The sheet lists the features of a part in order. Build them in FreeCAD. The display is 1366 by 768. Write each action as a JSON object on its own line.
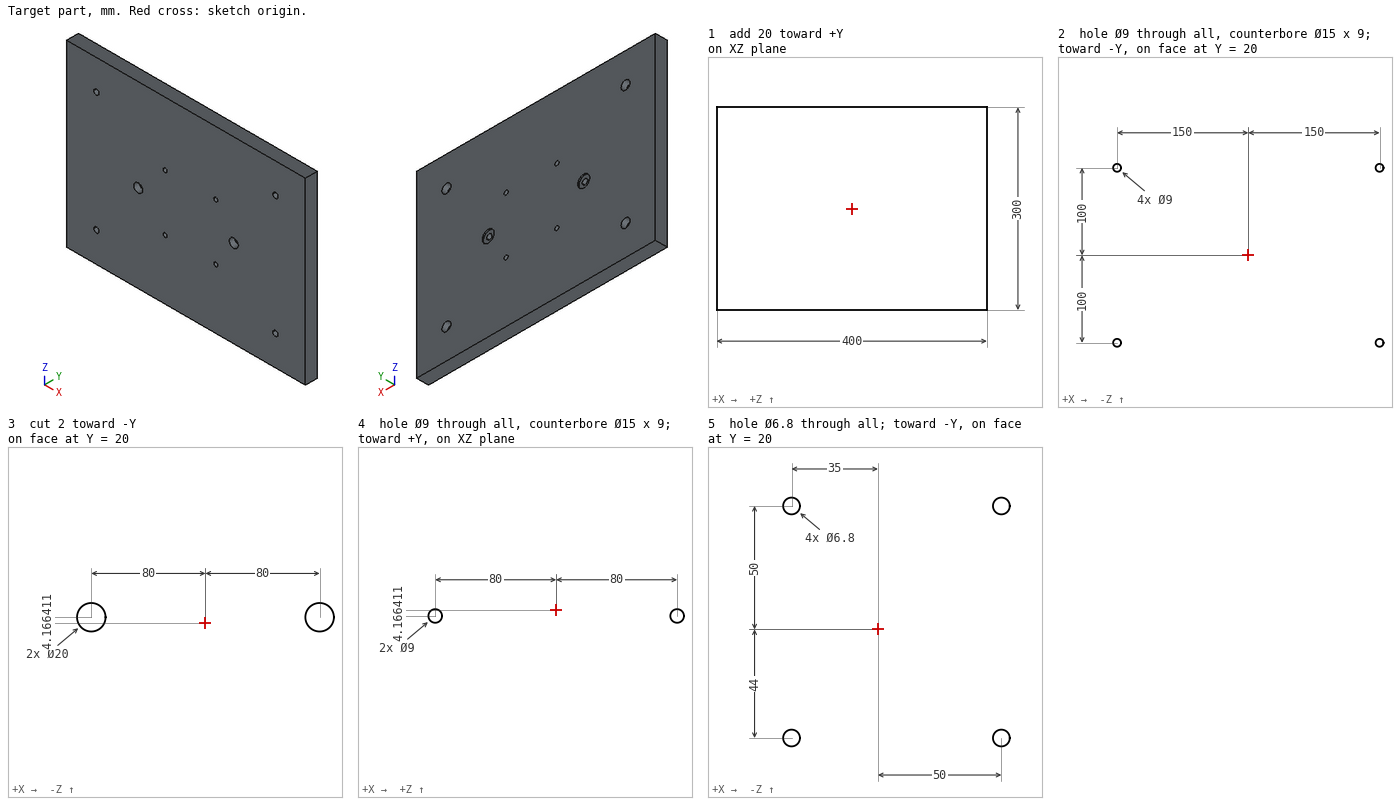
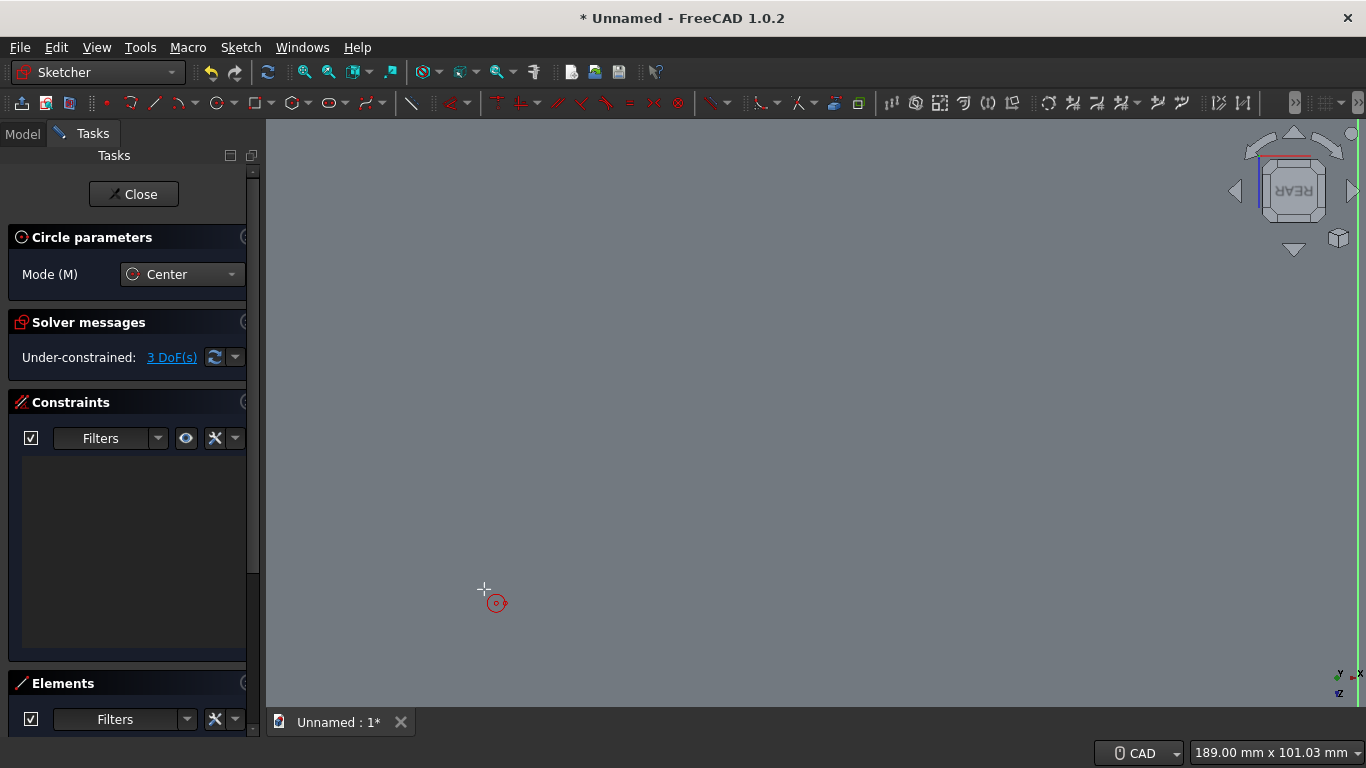
{"action": "left_click", "coordinate": [485, 586]}
{"action": "left_click", "coordinate": [503, 568]}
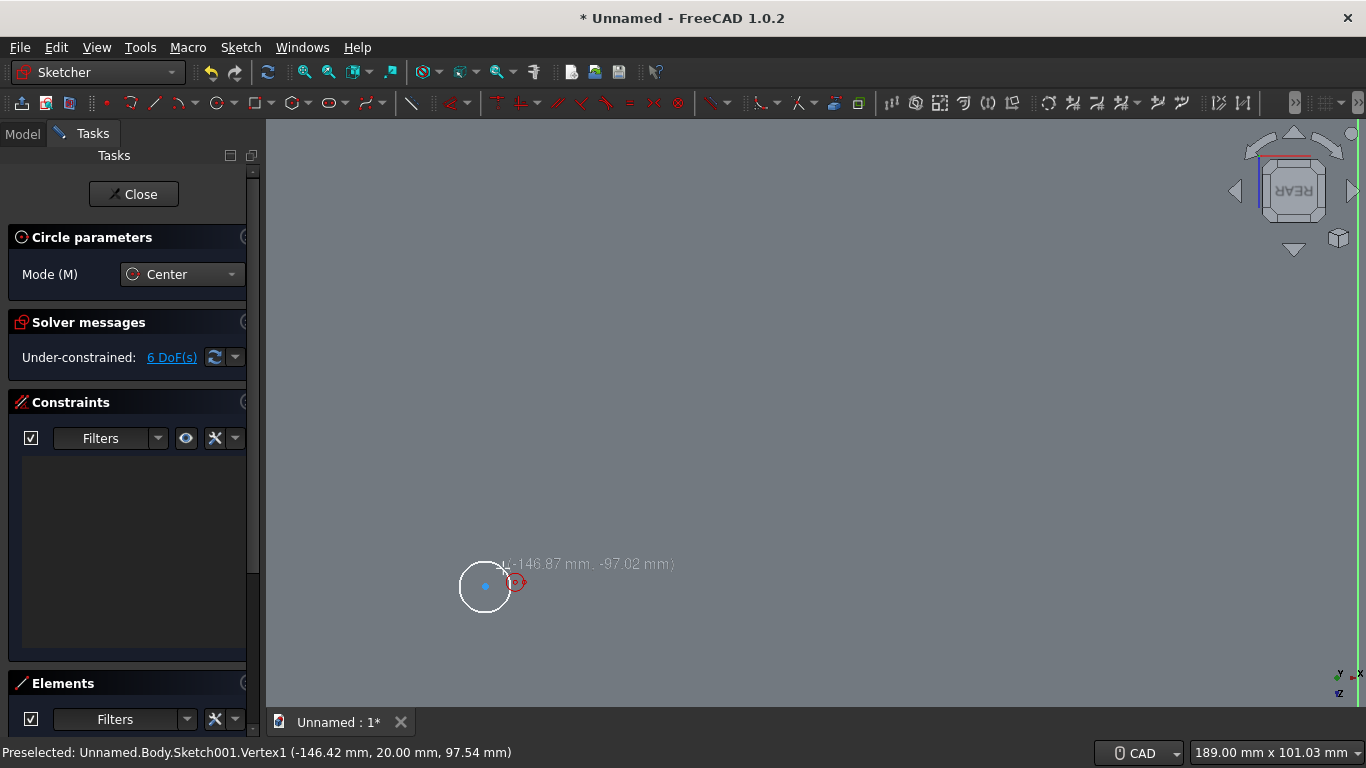
{"action": "scroll", "coordinate": [484, 589], "scroll_direction": "down", "scroll_amount": 6}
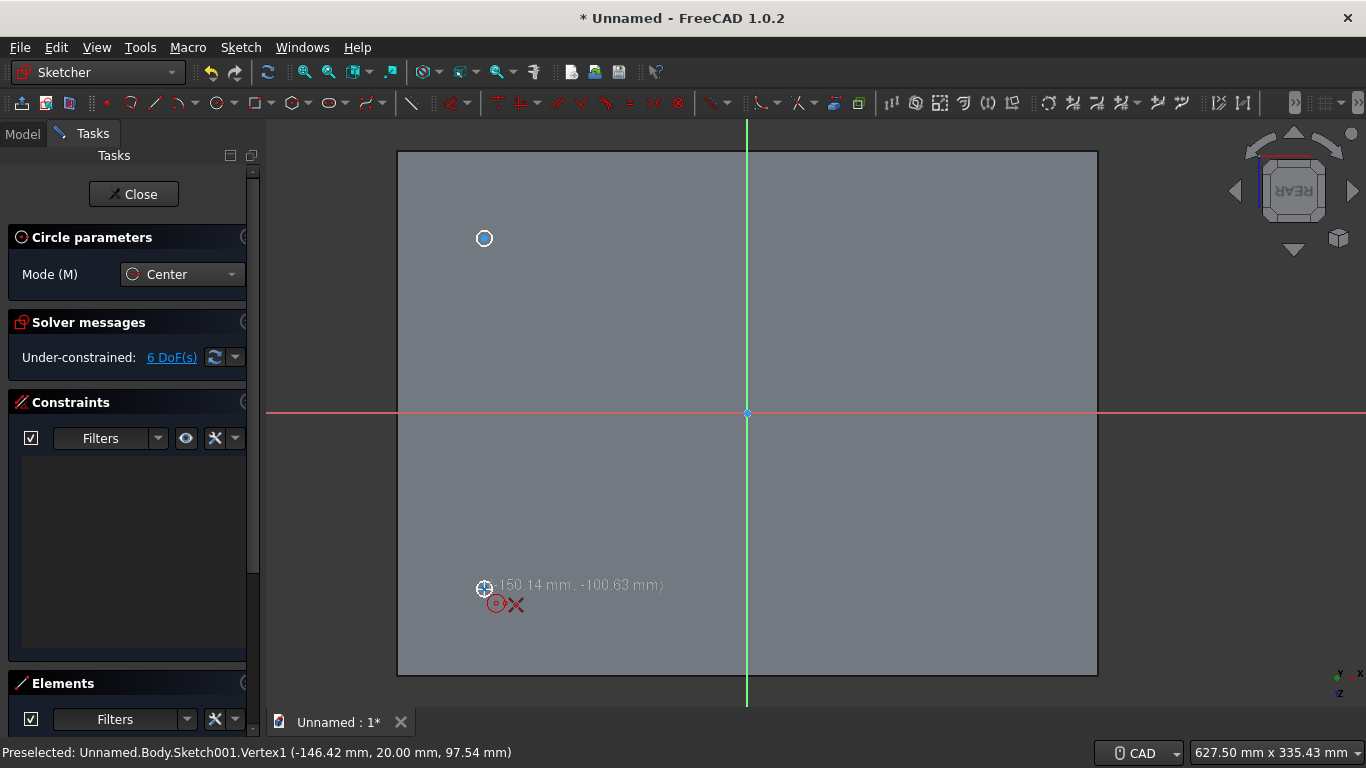
{"action": "scroll", "coordinate": [1010, 238], "scroll_direction": "up", "scroll_amount": 6}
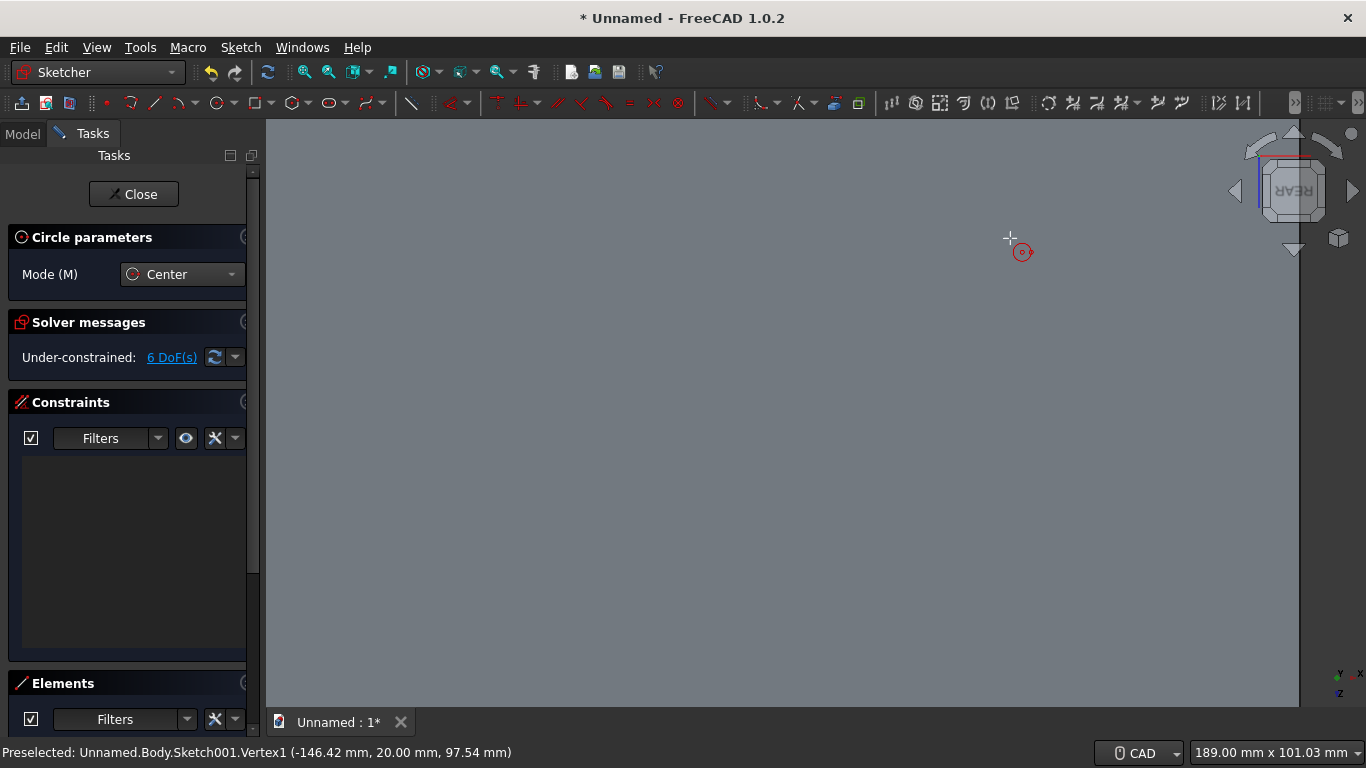
{"action": "left_click", "coordinate": [1009, 238]}
{"action": "left_click", "coordinate": [1028, 220]}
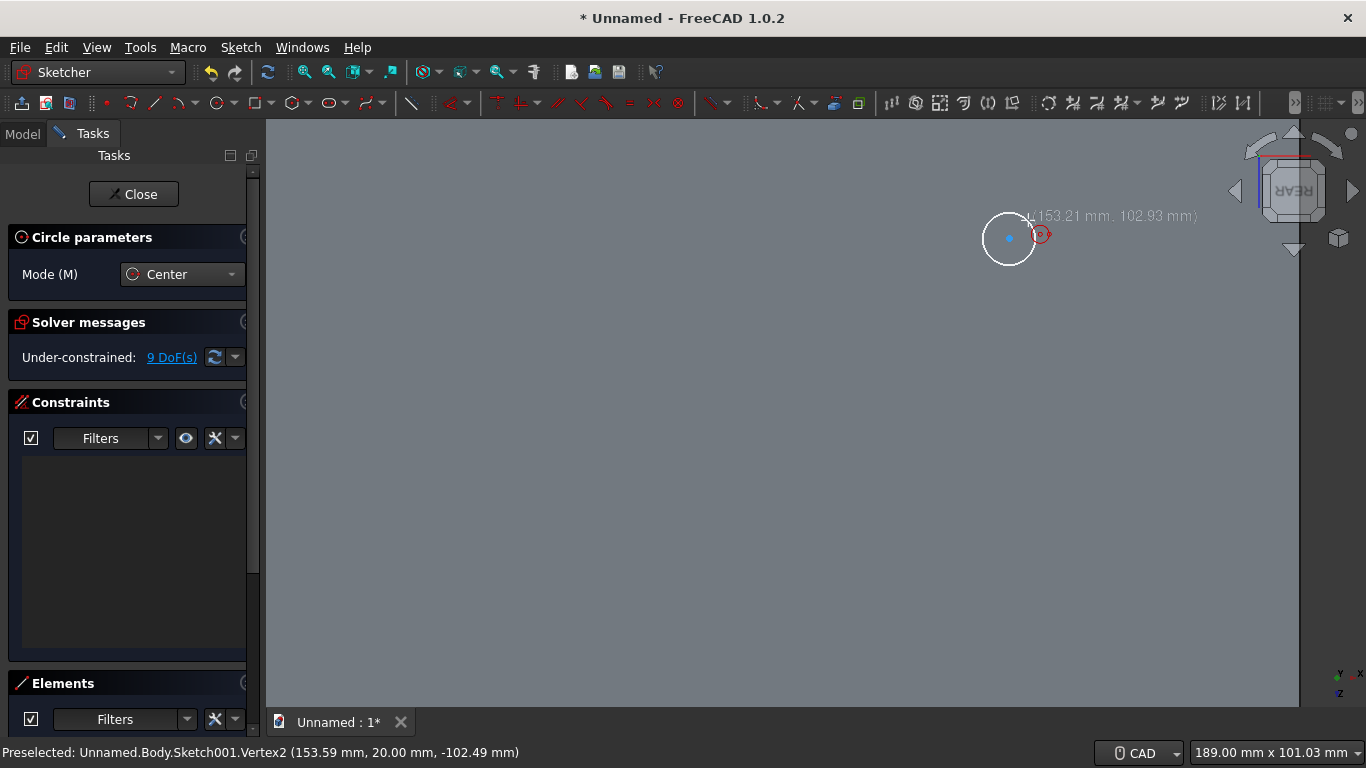
{"action": "scroll", "coordinate": [1011, 238], "scroll_direction": "down", "scroll_amount": 6}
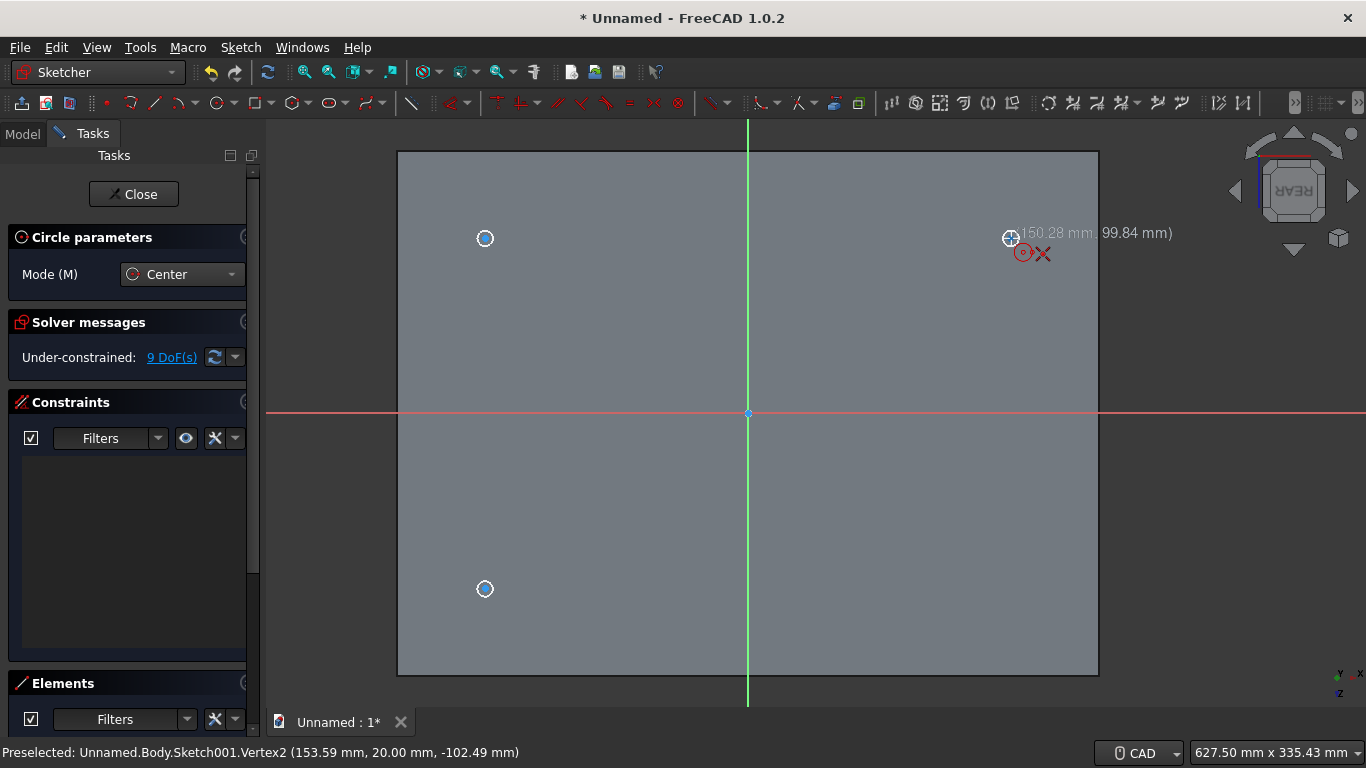
{"action": "scroll", "coordinate": [1011, 589], "scroll_direction": "up", "scroll_amount": 6}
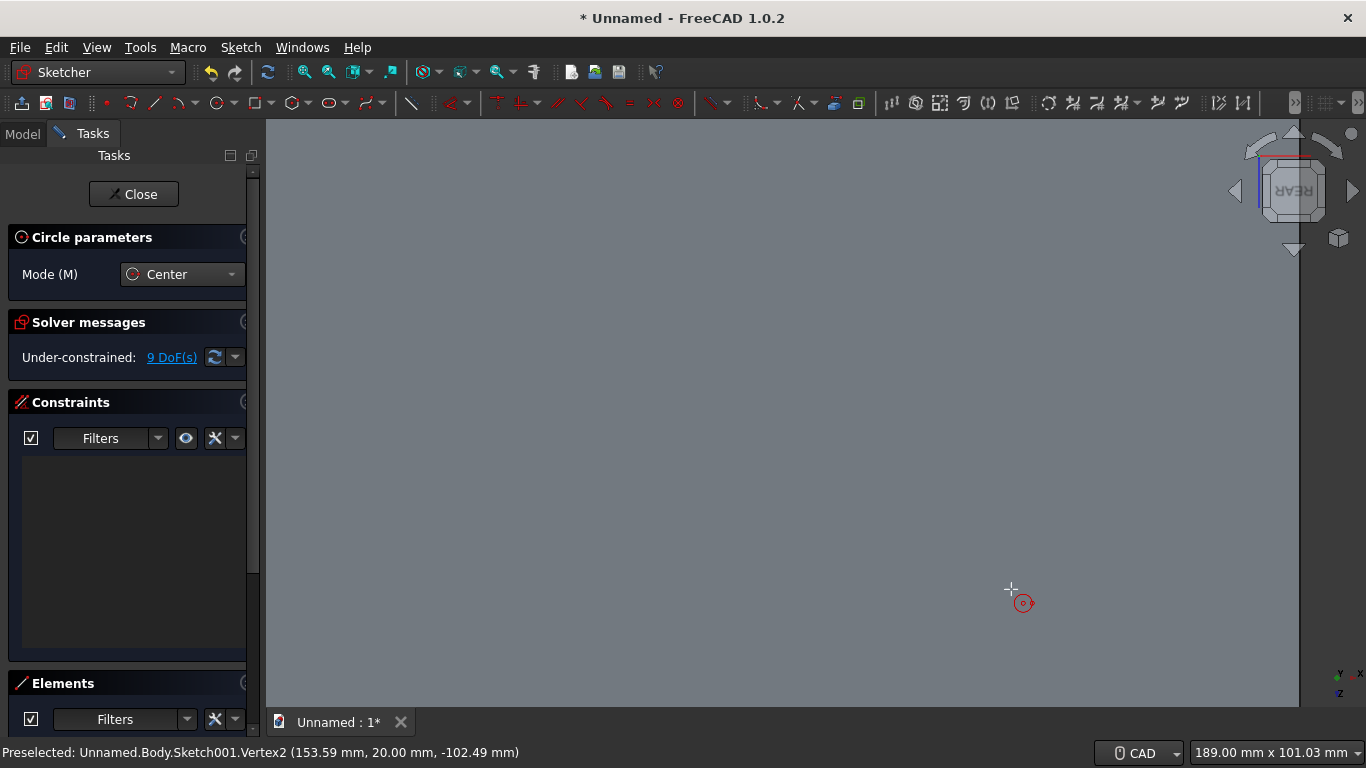
{"action": "left_click", "coordinate": [1009, 586]}
{"action": "left_click", "coordinate": [1028, 568]}
{"action": "key", "text": "Escape"}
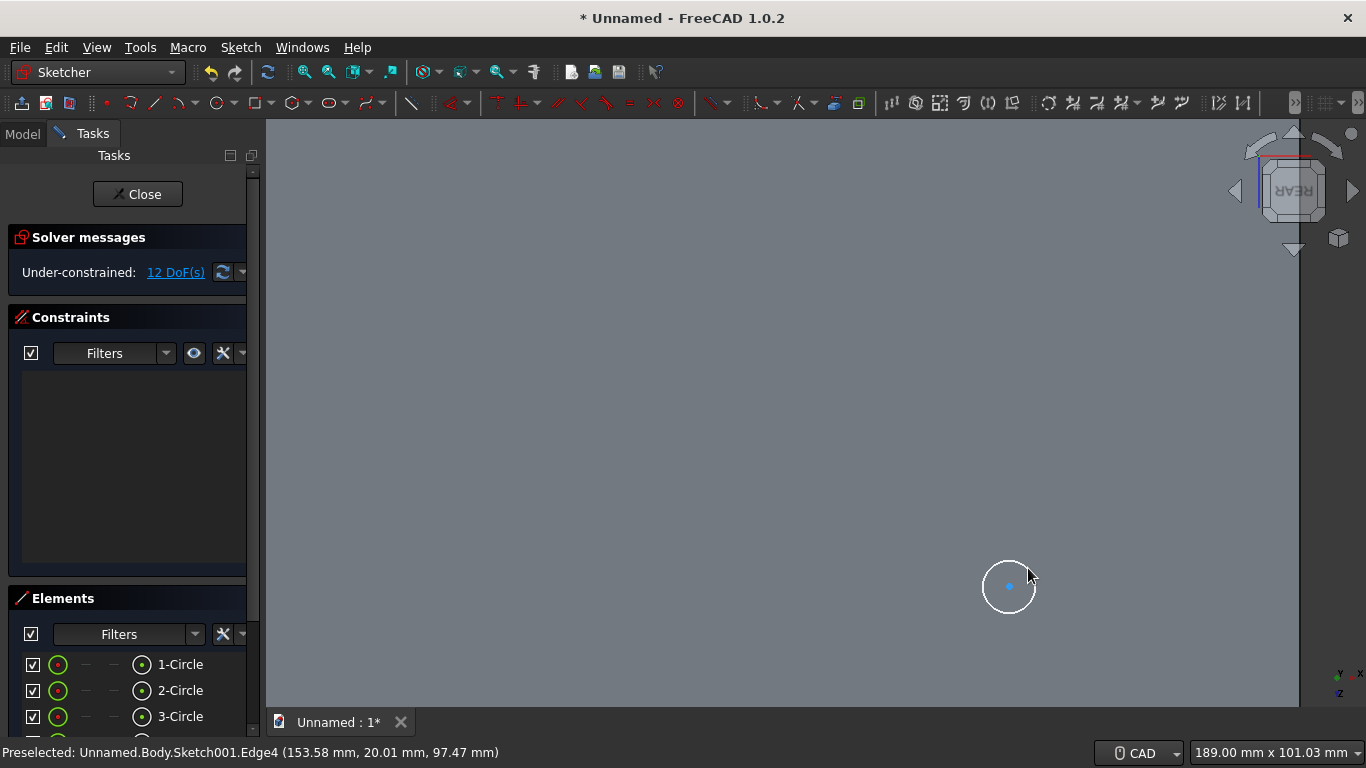
{"action": "scroll", "coordinate": [1011, 589], "scroll_direction": "down", "scroll_amount": 6}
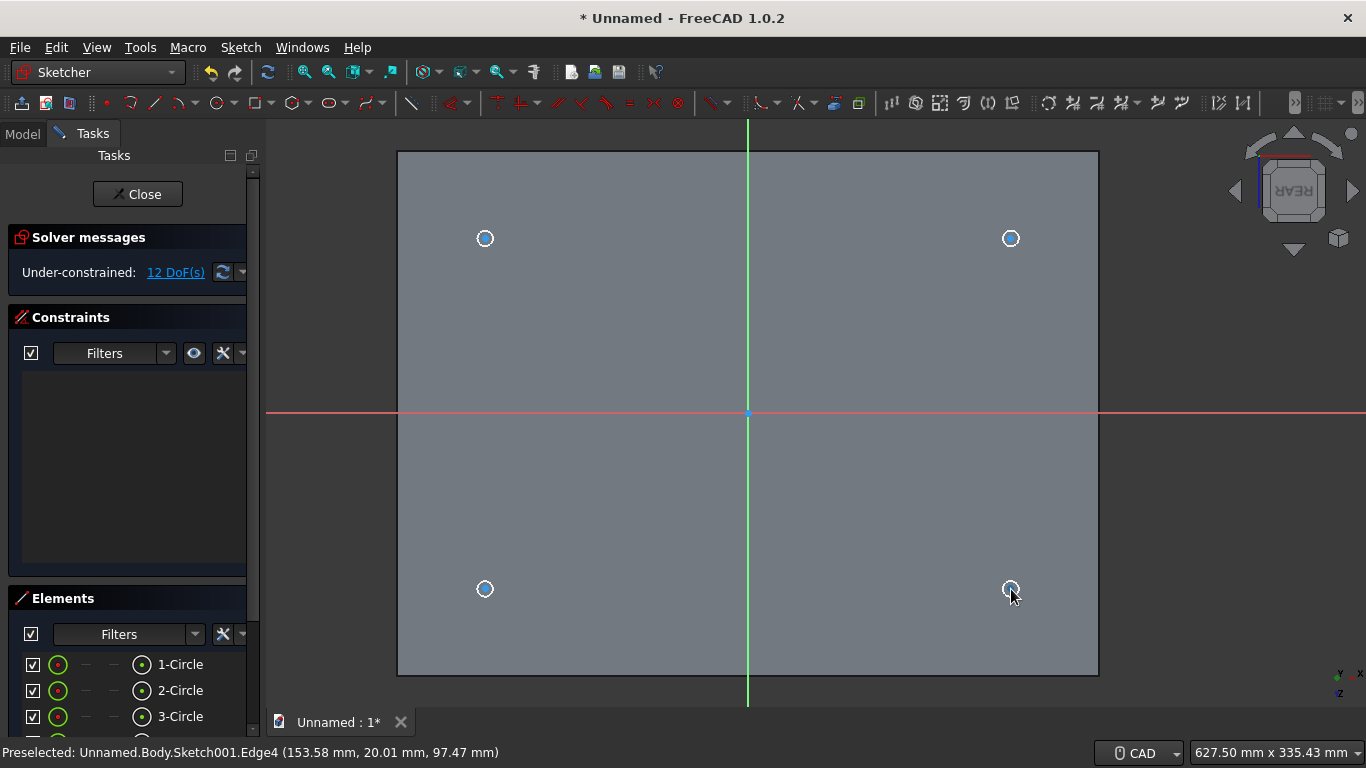
{"action": "scroll", "coordinate": [491, 233], "scroll_direction": "up", "scroll_amount": 3}